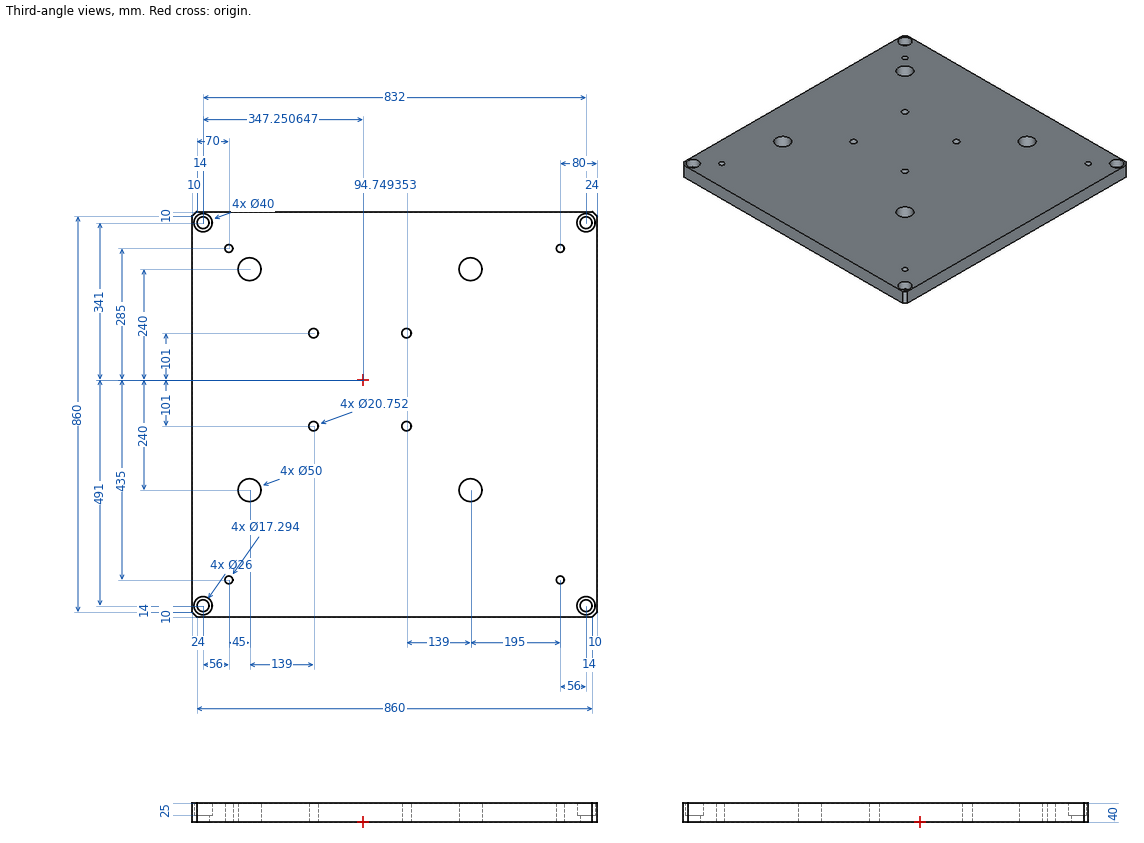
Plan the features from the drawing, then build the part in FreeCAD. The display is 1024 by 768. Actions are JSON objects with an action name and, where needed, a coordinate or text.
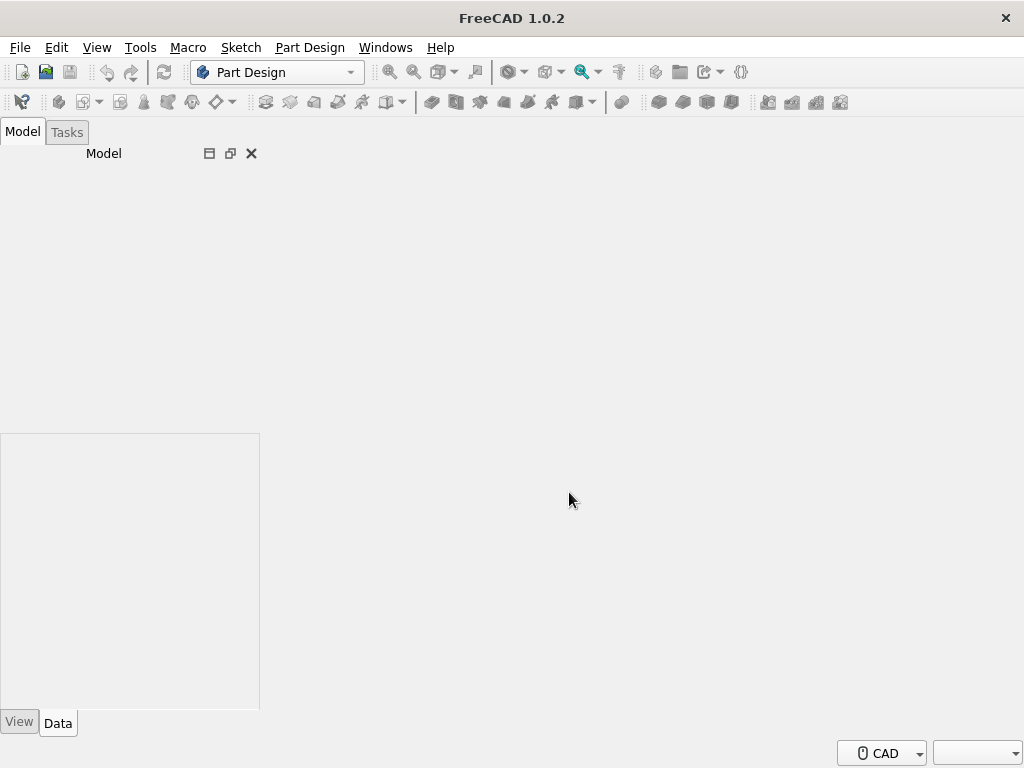
{"action": "left_click", "coordinate": [22, 72]}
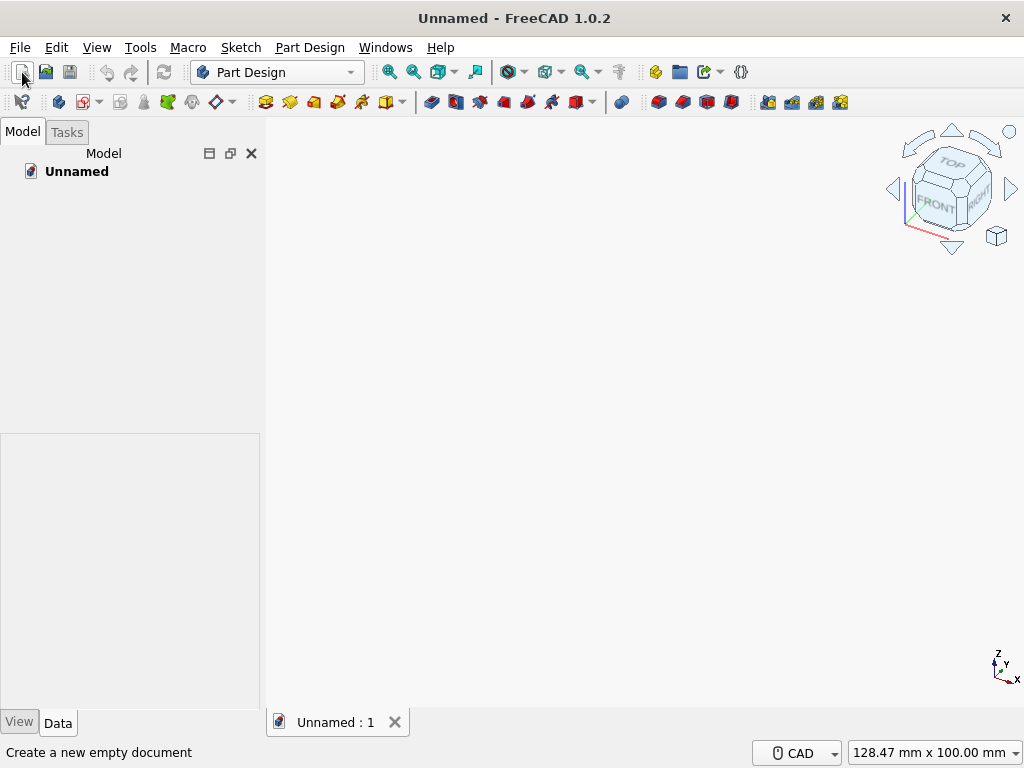
{"action": "left_click", "coordinate": [84, 102]}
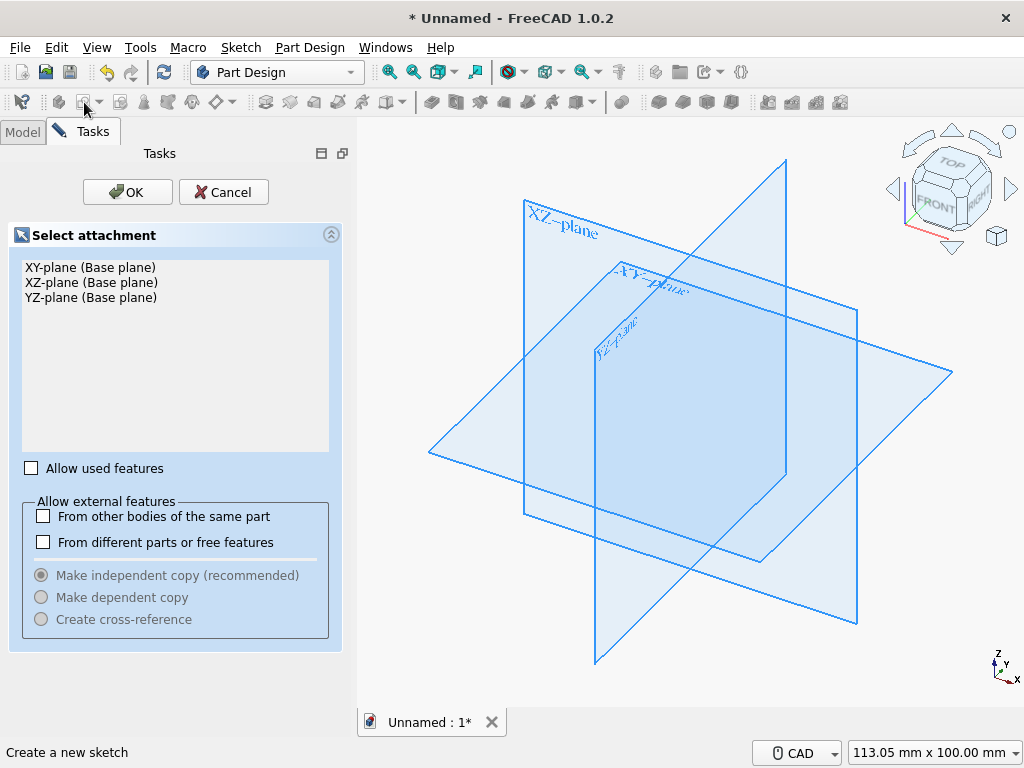
{"action": "left_click", "coordinate": [82, 268]}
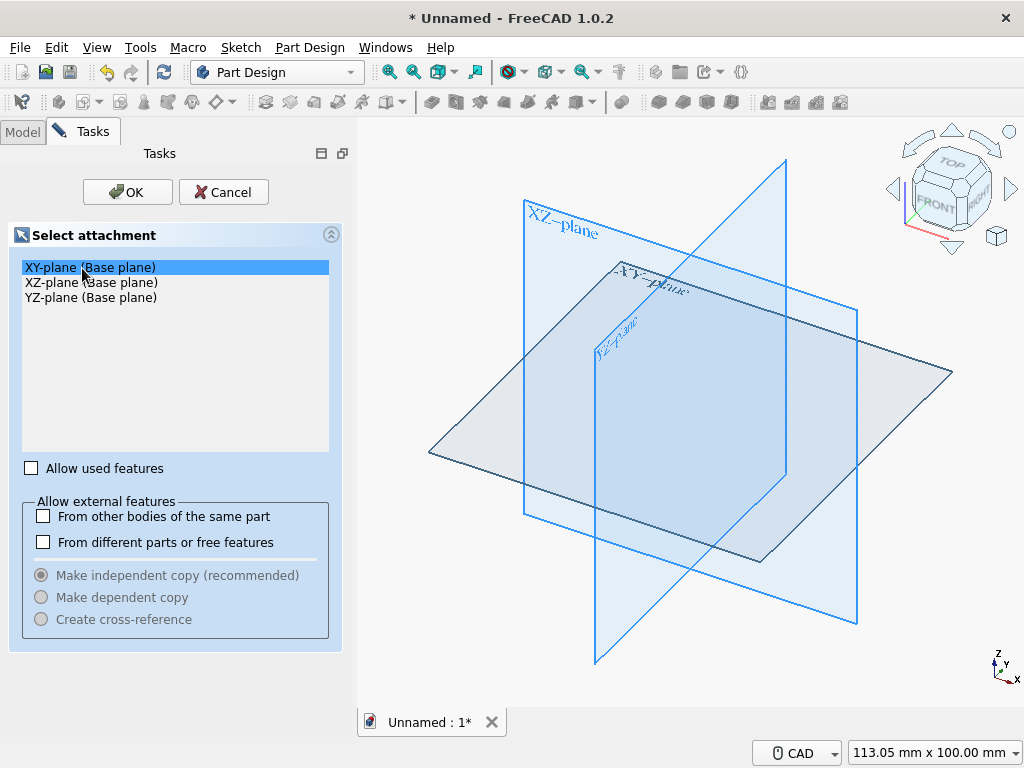
{"action": "left_click", "coordinate": [128, 192]}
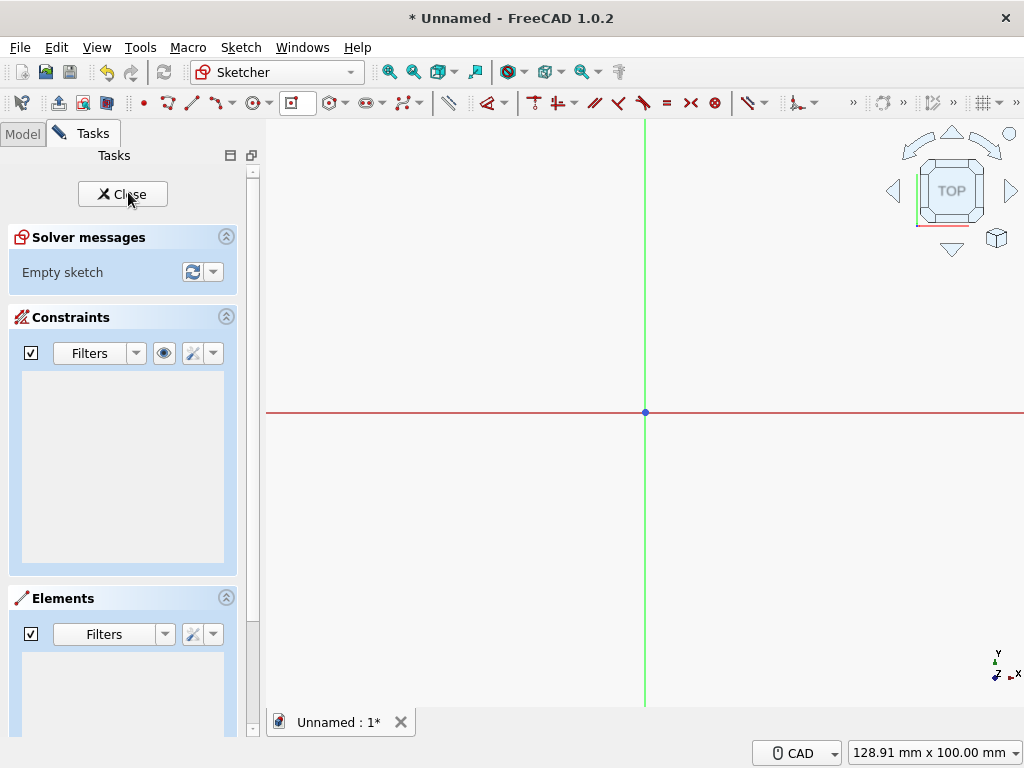
{"action": "scroll", "coordinate": [539, 378], "scroll_direction": "down", "scroll_amount": 13}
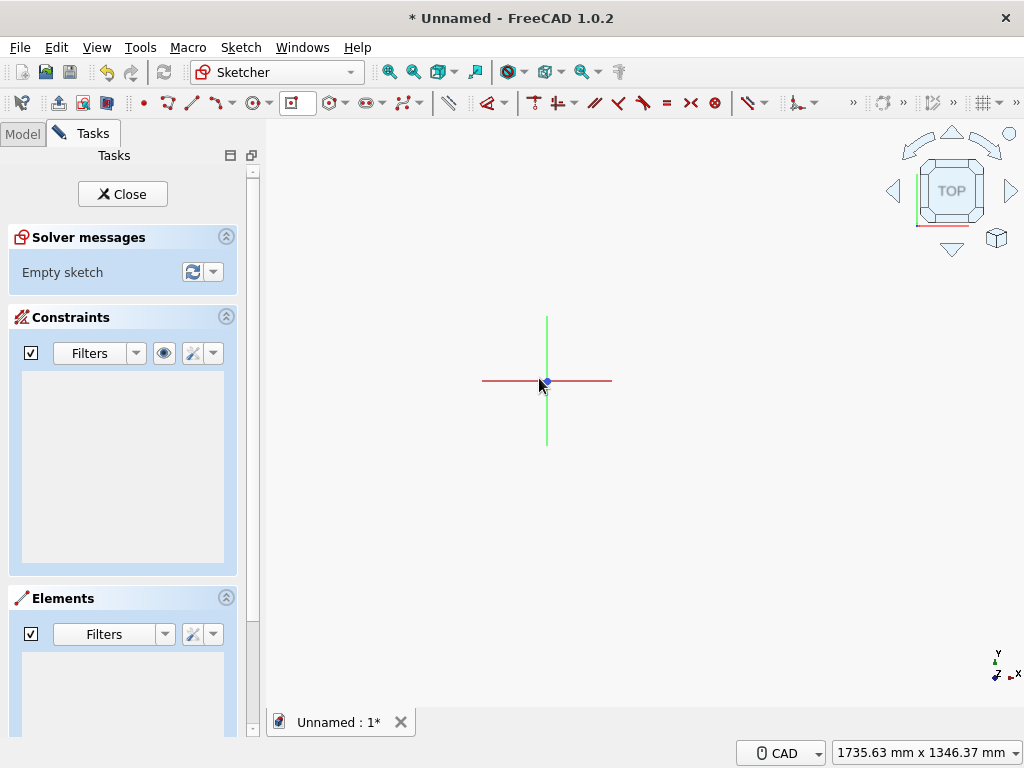
{"action": "key", "text": "g m"}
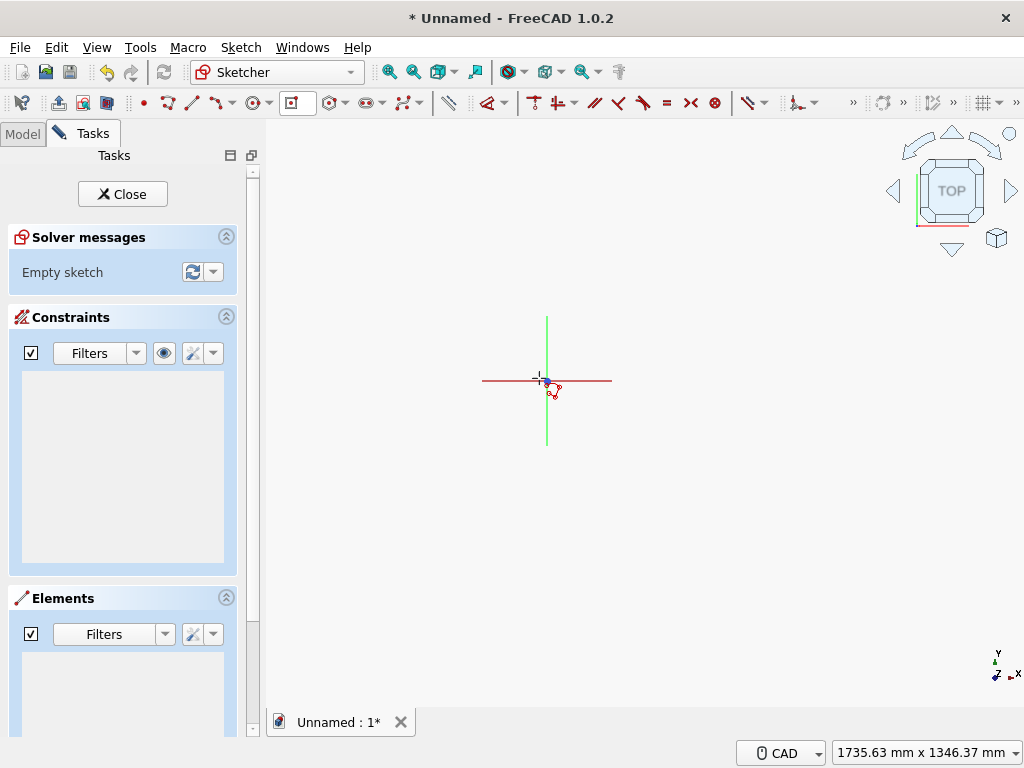
{"action": "left_click", "coordinate": [389, 222]}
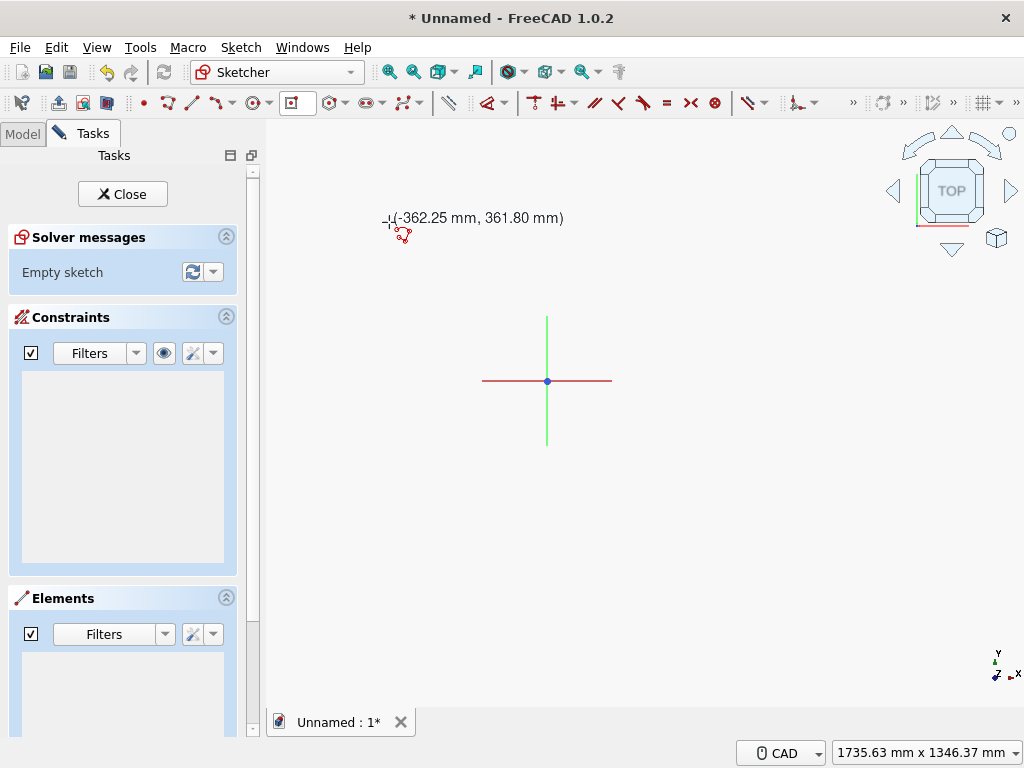
{"action": "scroll", "coordinate": [385, 226], "scroll_direction": "up", "scroll_amount": 5}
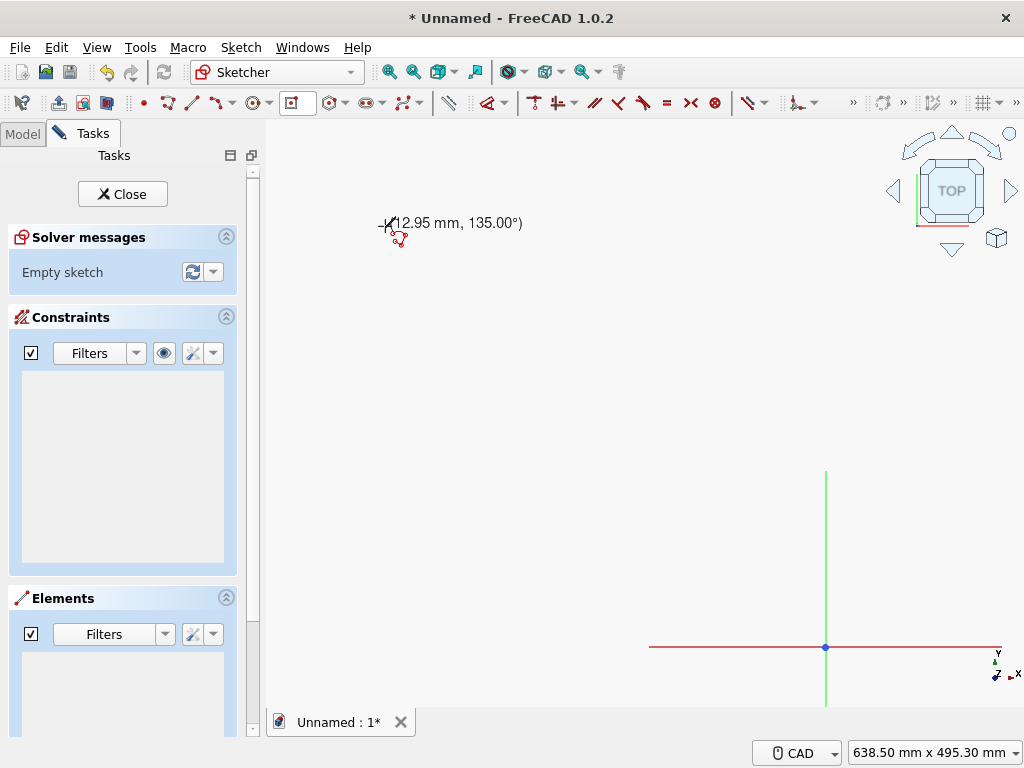
{"action": "left_click", "coordinate": [385, 226]}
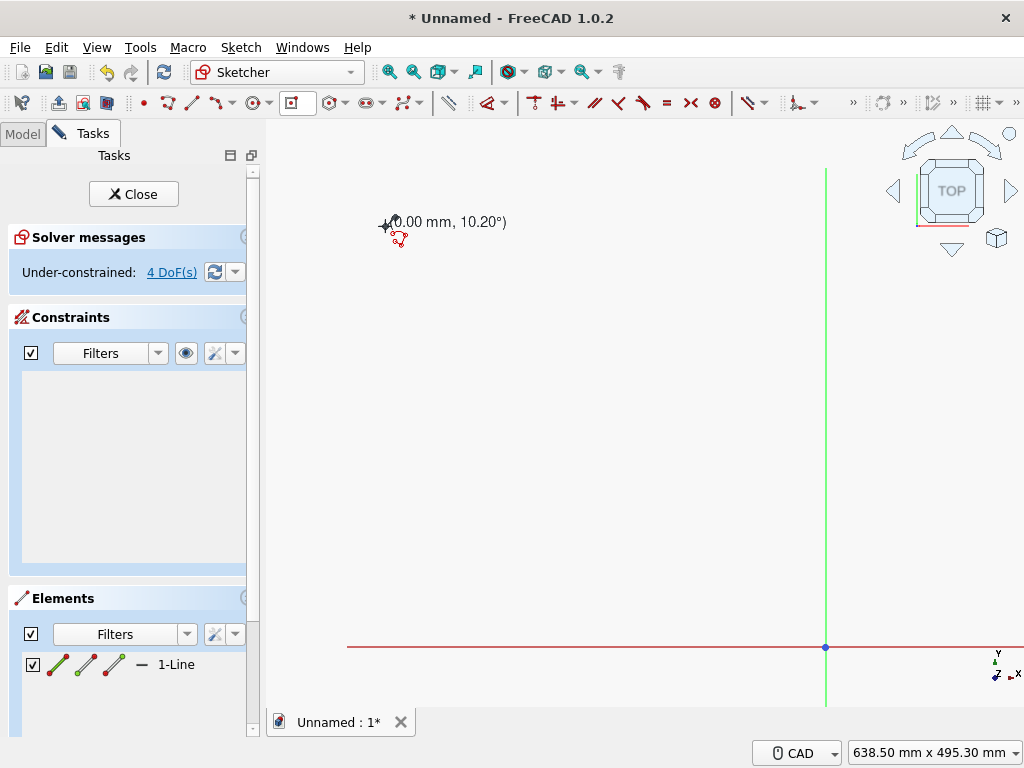
{"action": "scroll", "coordinate": [384, 225], "scroll_direction": "down", "scroll_amount": 5}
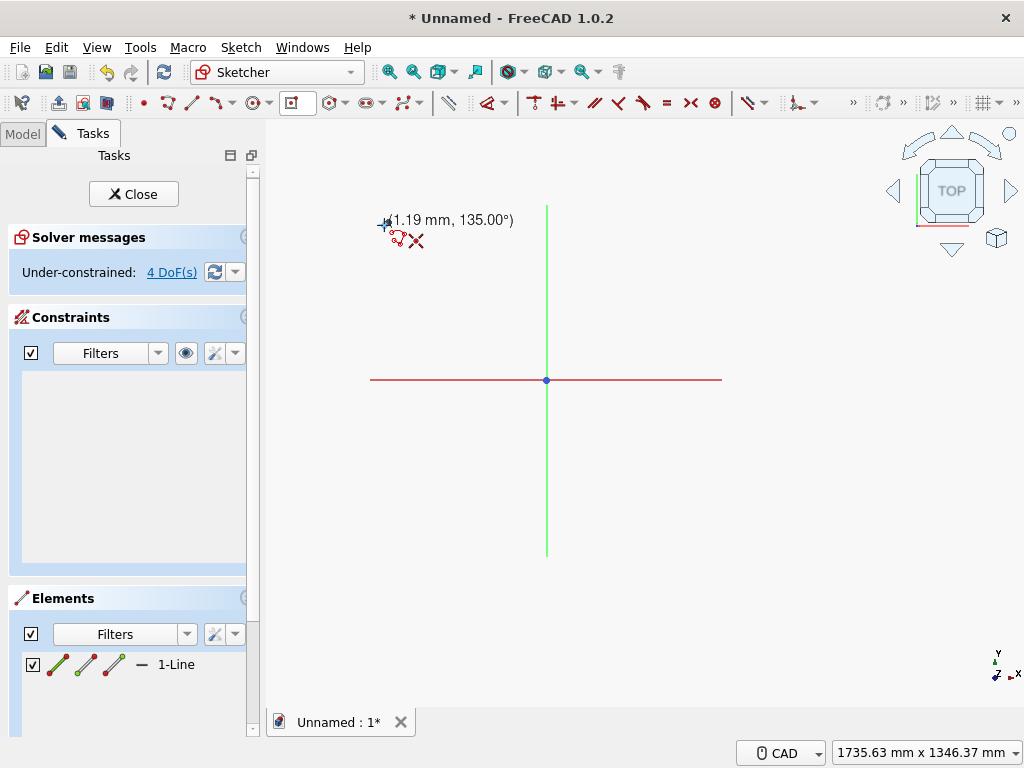
{"action": "left_click", "coordinate": [384, 601]}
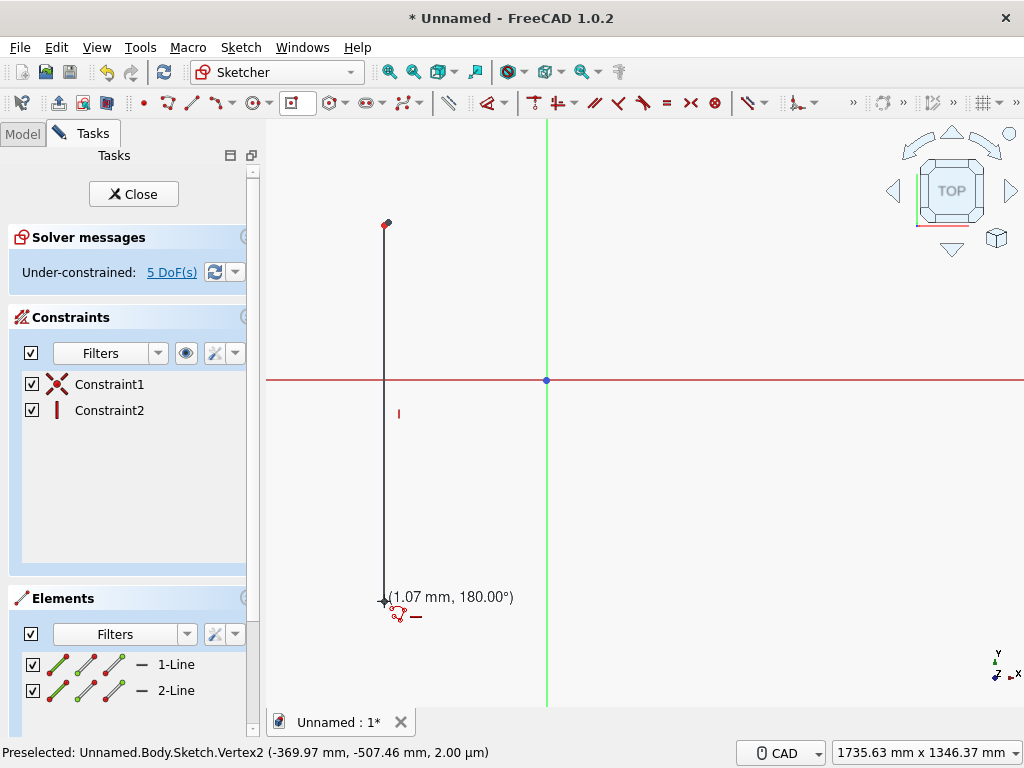
{"action": "scroll", "coordinate": [389, 605], "scroll_direction": "up", "scroll_amount": 5}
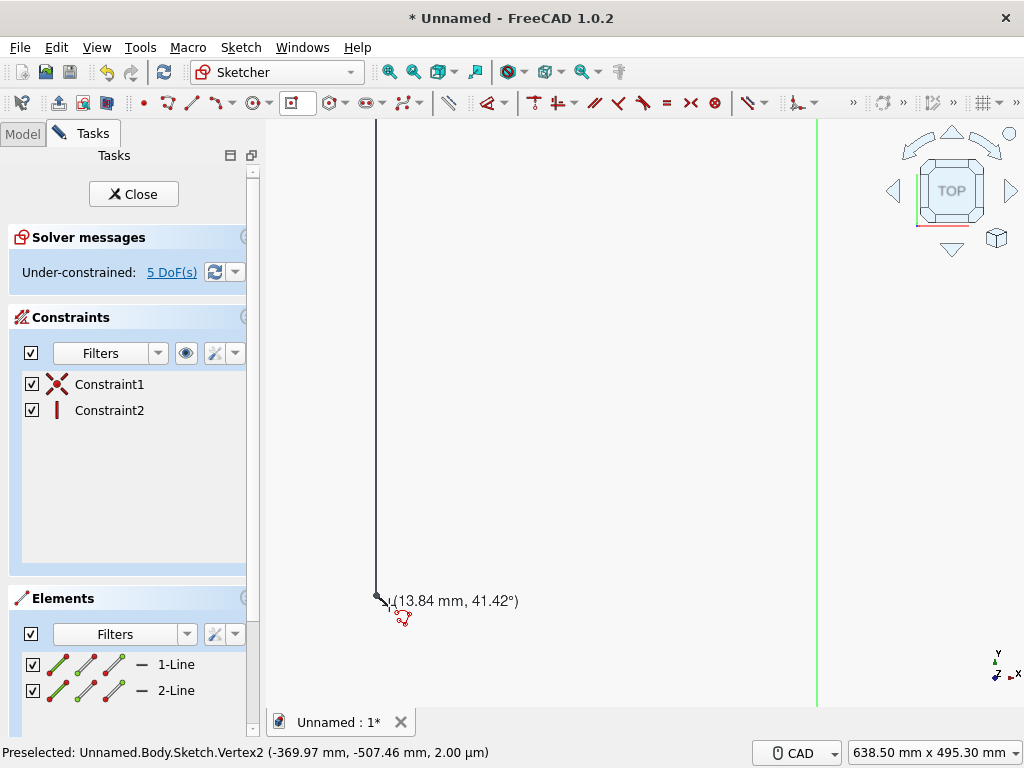
{"action": "left_click", "coordinate": [388, 604]}